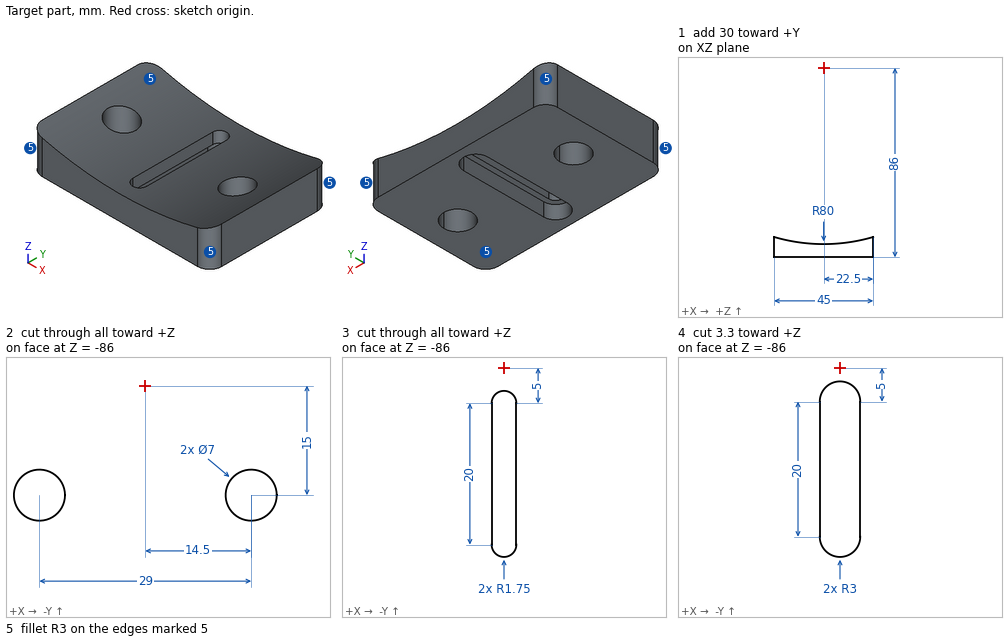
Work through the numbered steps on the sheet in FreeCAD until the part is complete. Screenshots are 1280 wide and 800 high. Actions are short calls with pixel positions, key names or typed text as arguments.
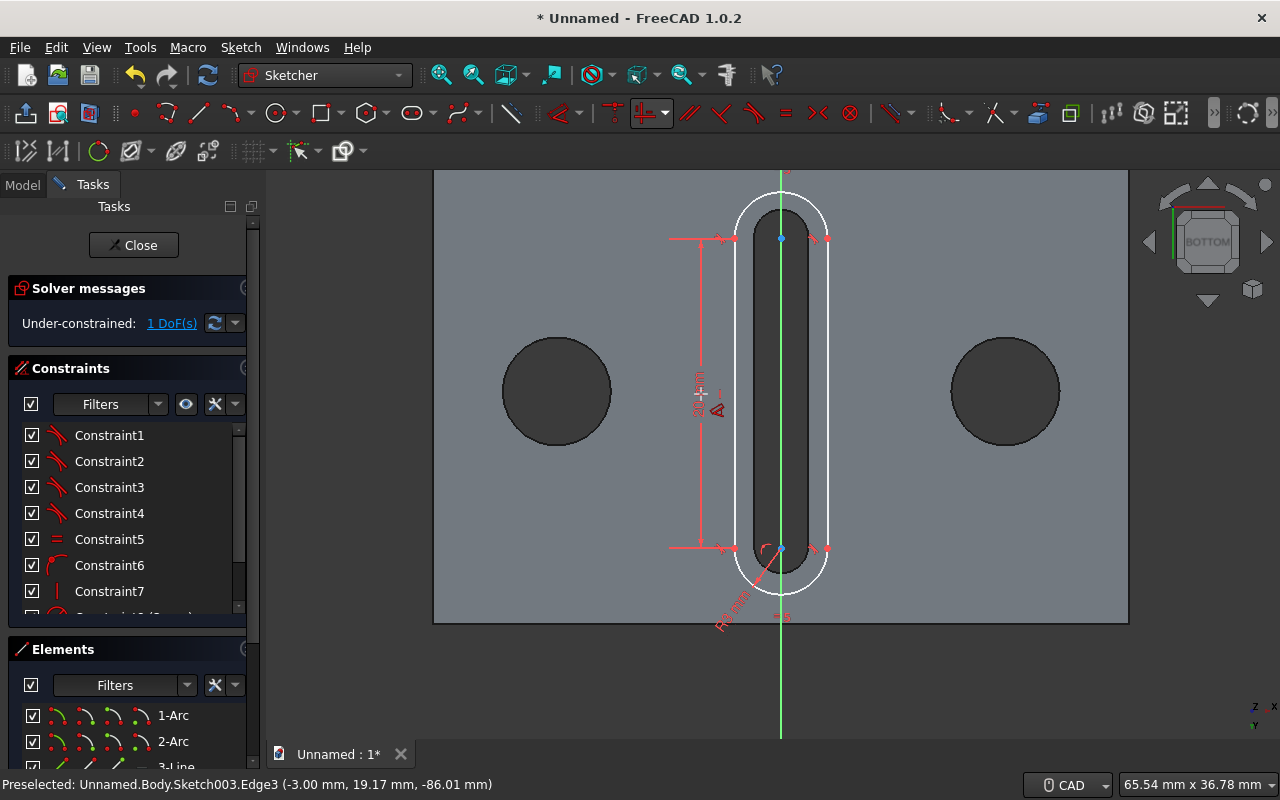
click(828, 239)
click(862, 218)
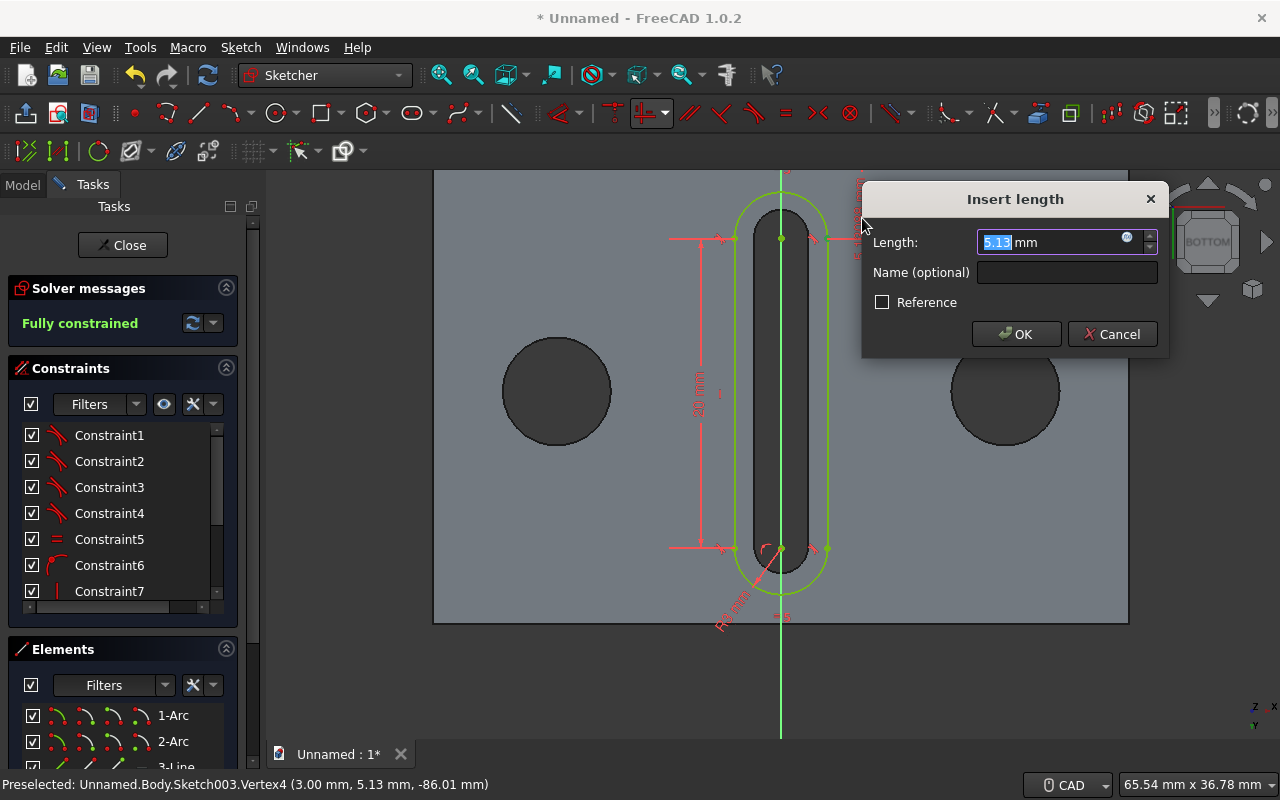
text(5)
key(Return)
key(Escape)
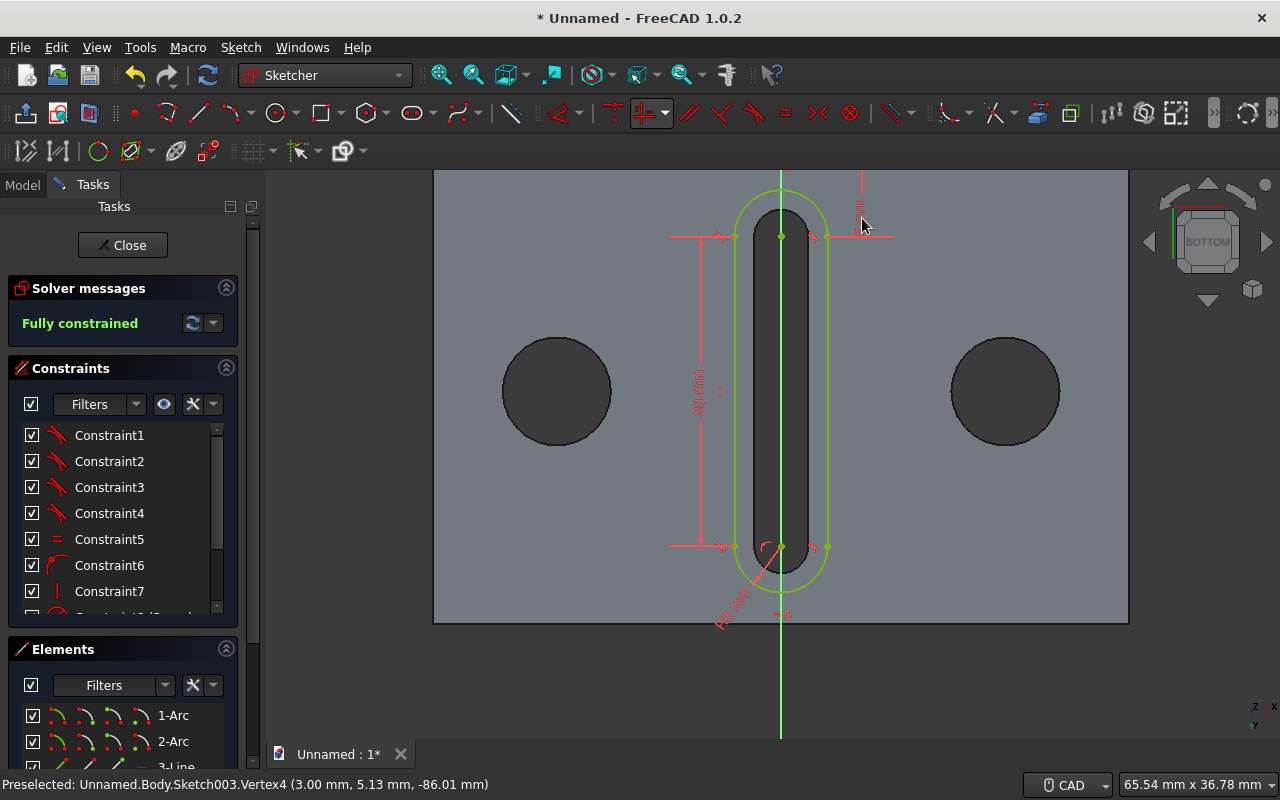
click(123, 245)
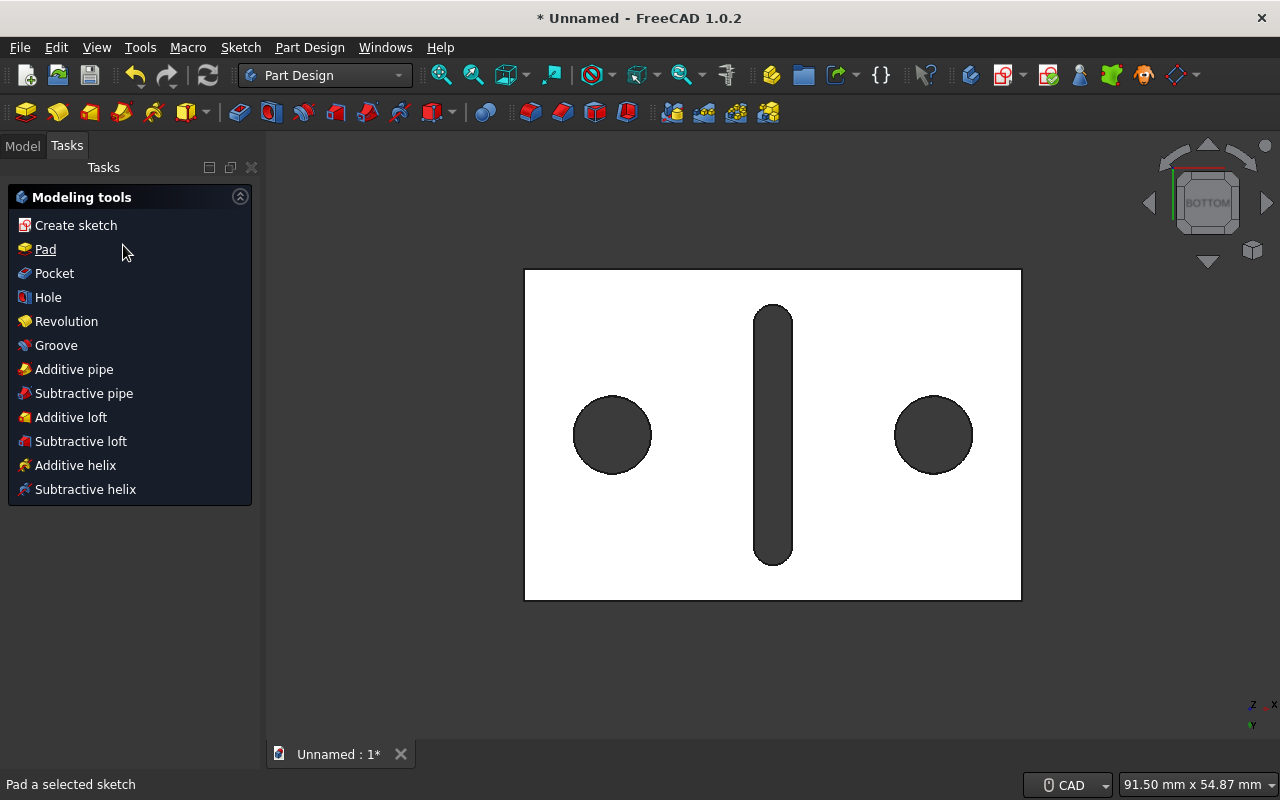
click(240, 112)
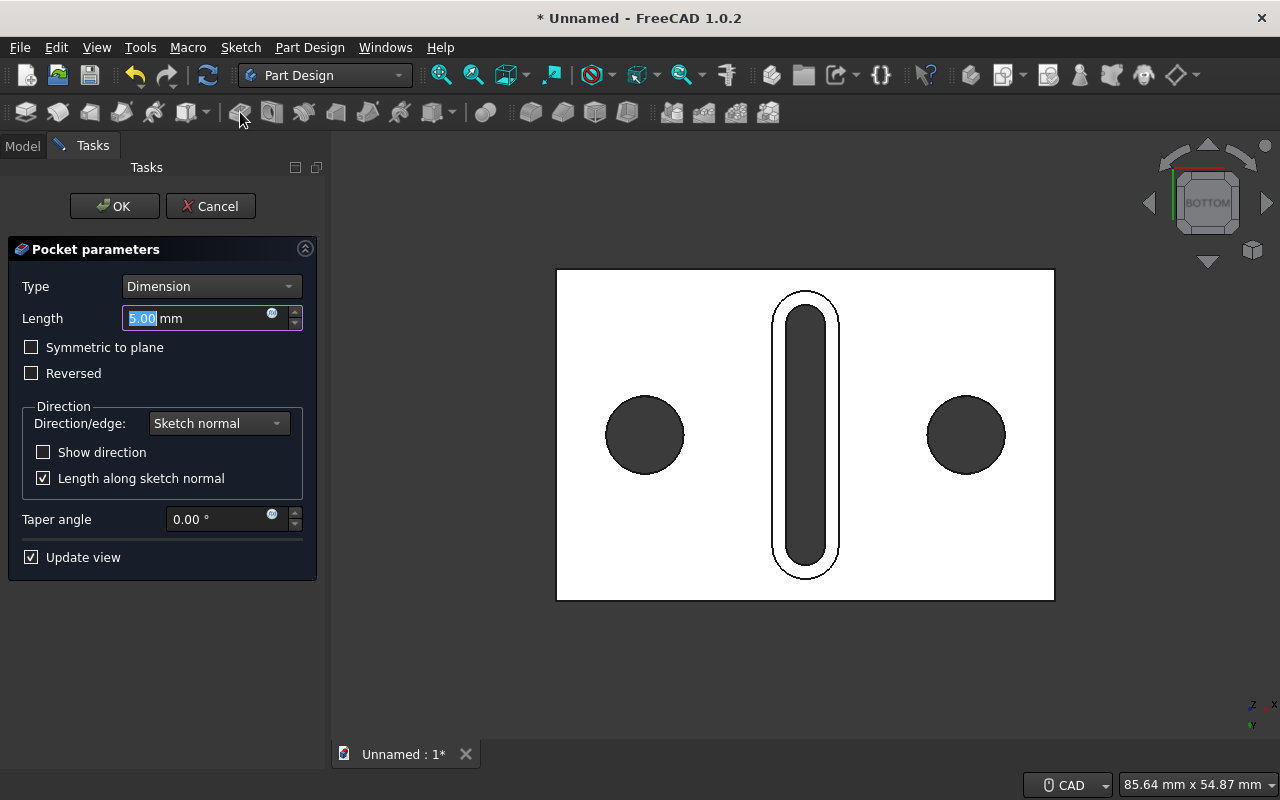
text(3.3)
key(Tab)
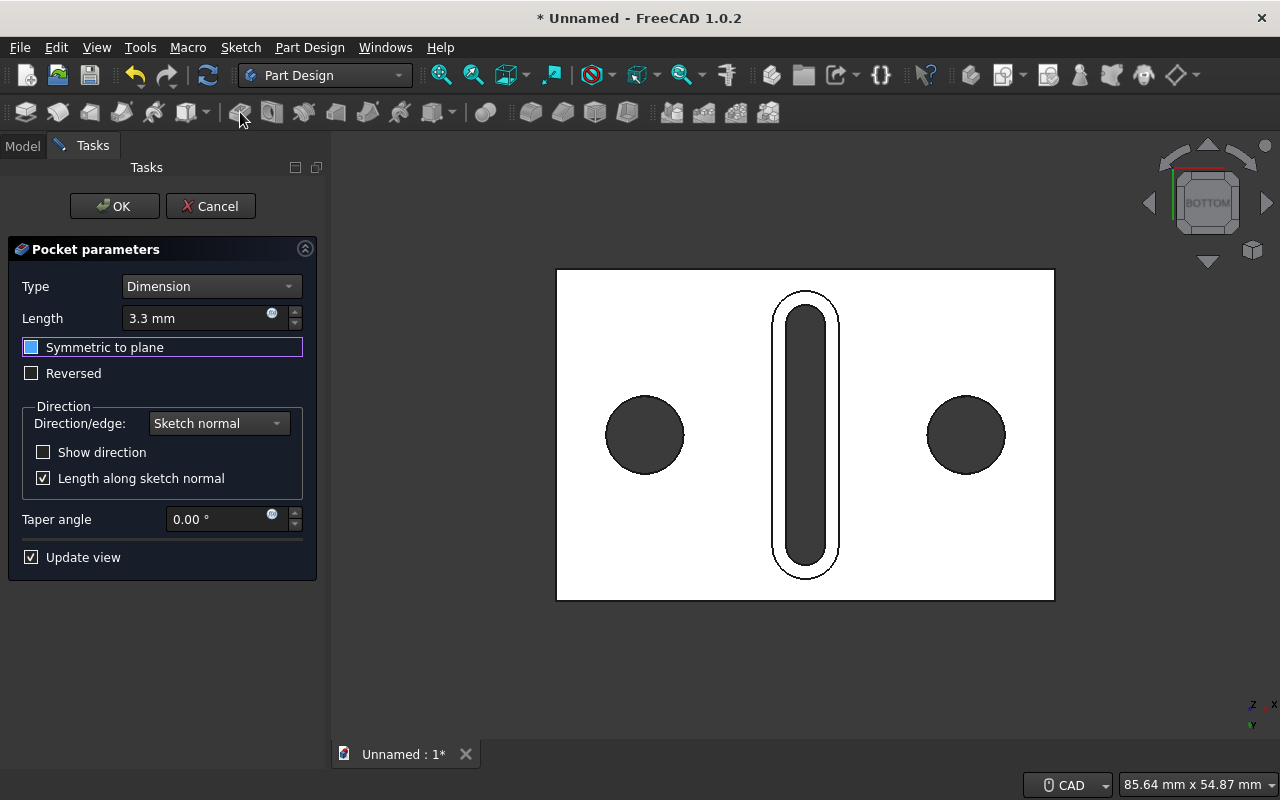
click(115, 206)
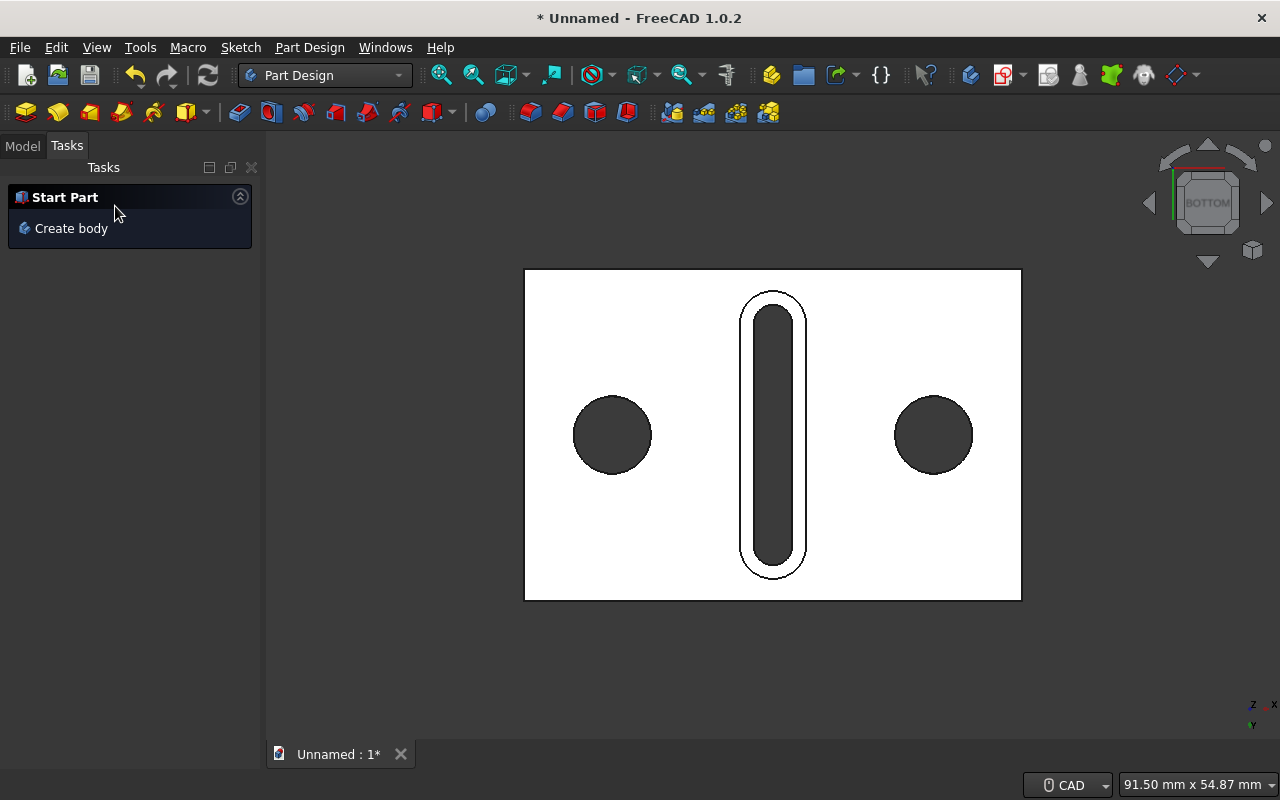
key(0)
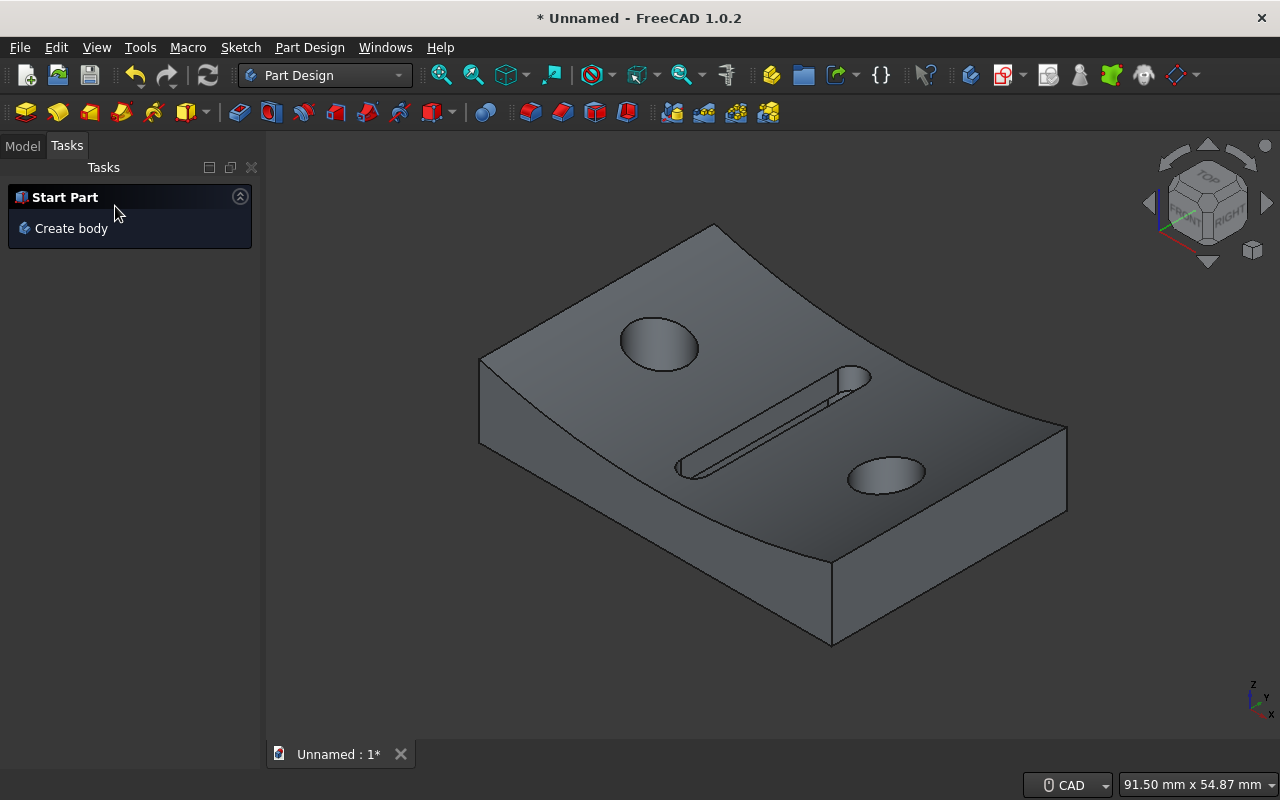
click(832, 604)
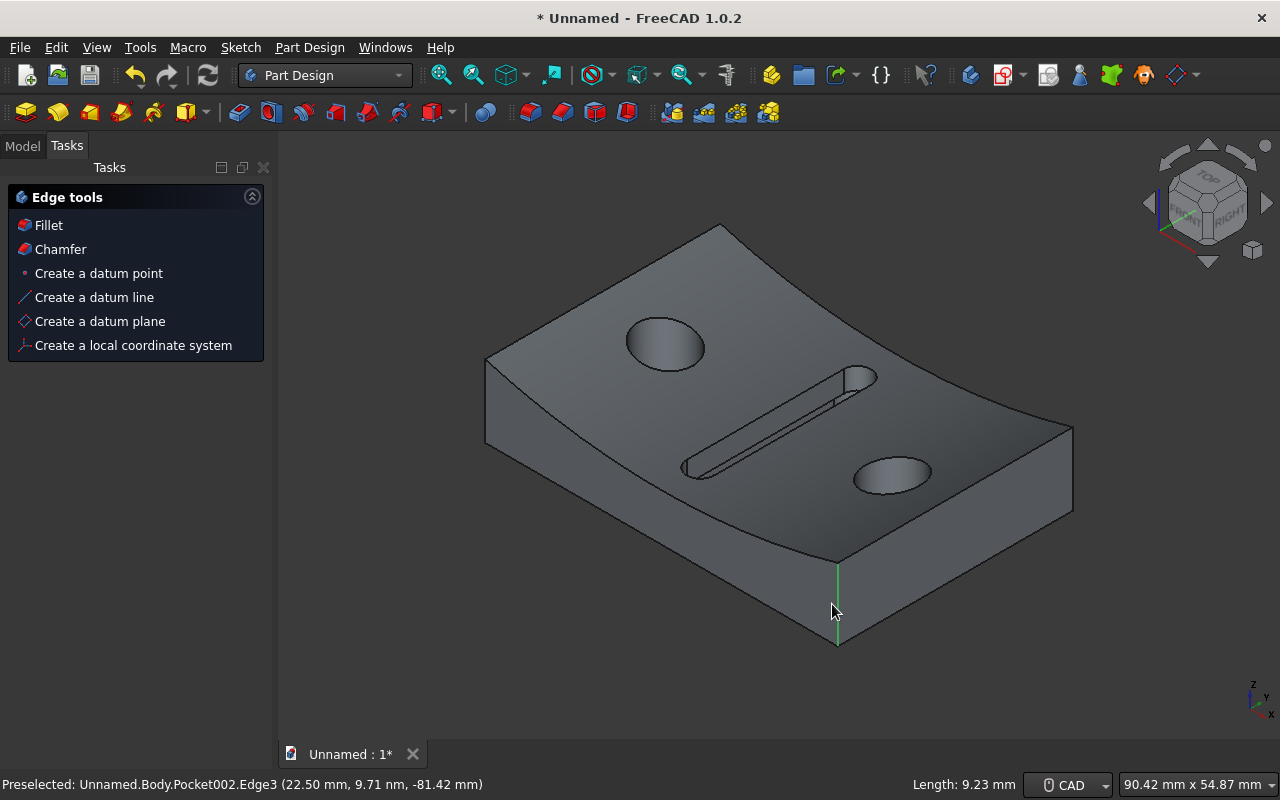
key(2)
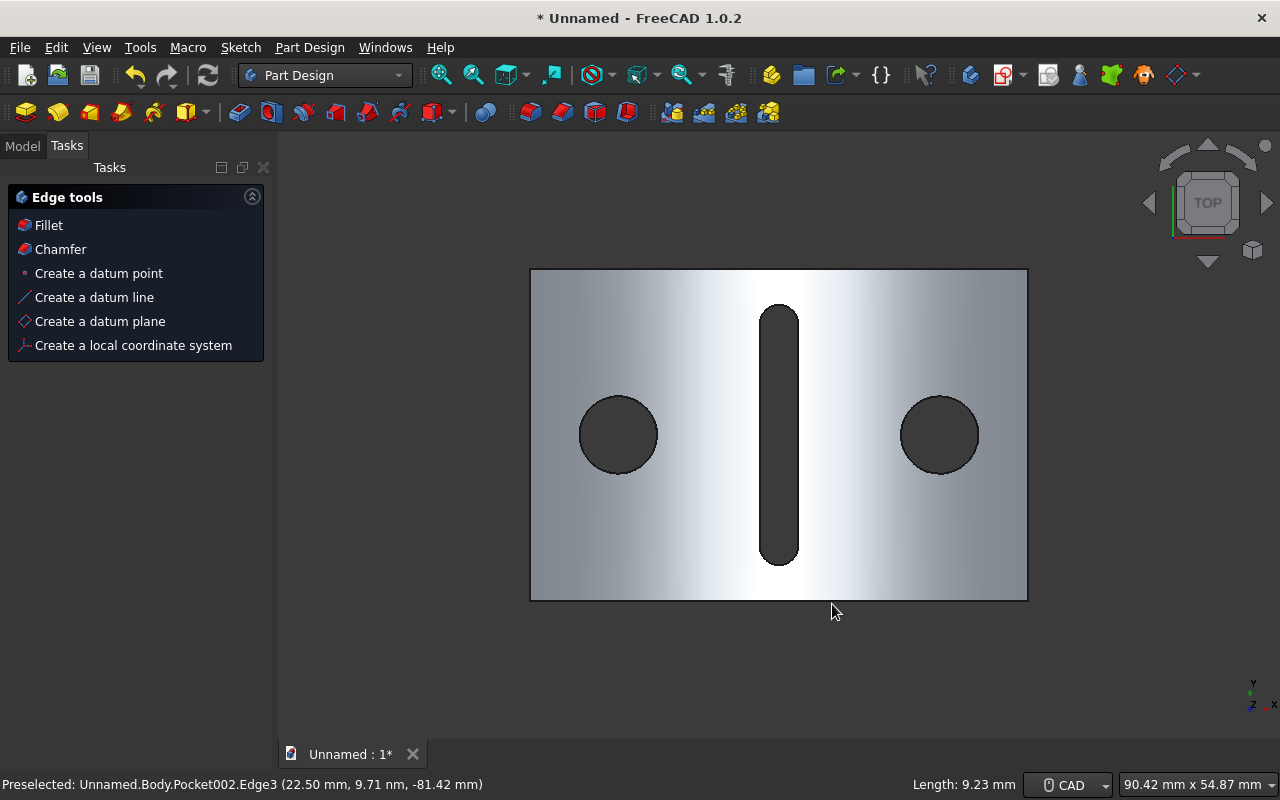
key(1)